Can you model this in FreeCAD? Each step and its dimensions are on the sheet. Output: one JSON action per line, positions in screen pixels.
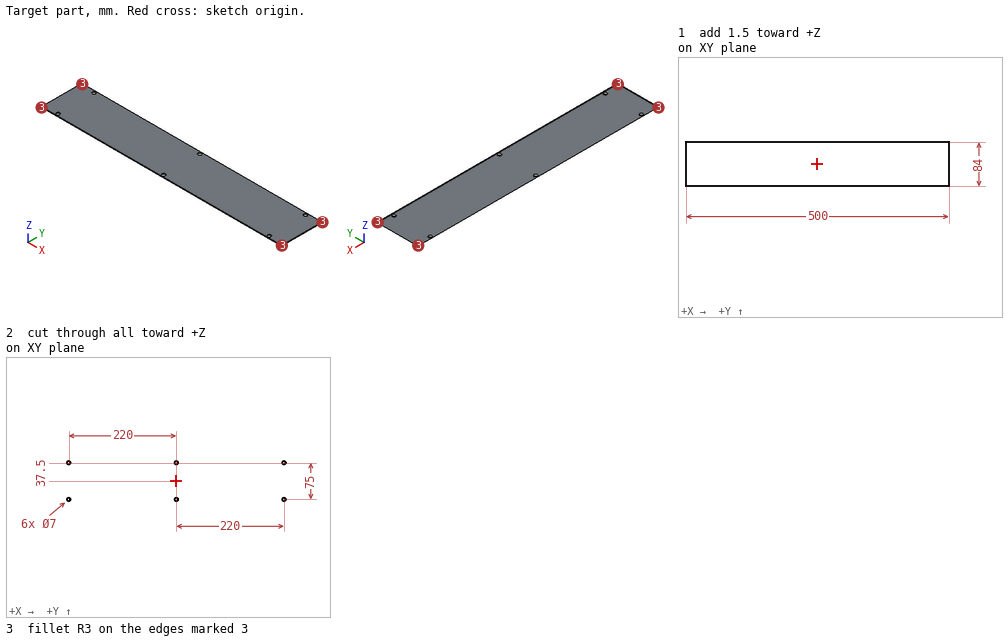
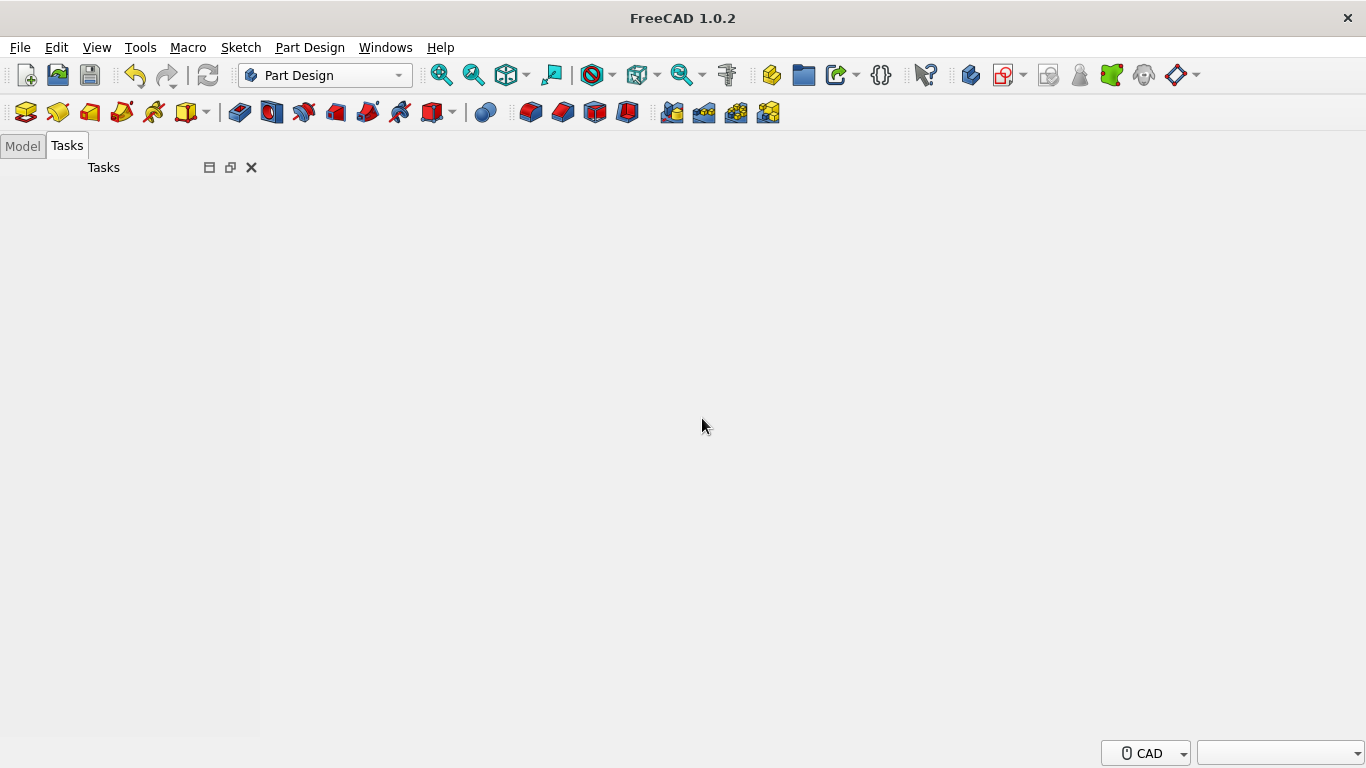
{"action": "left_click", "coordinate": [26, 76]}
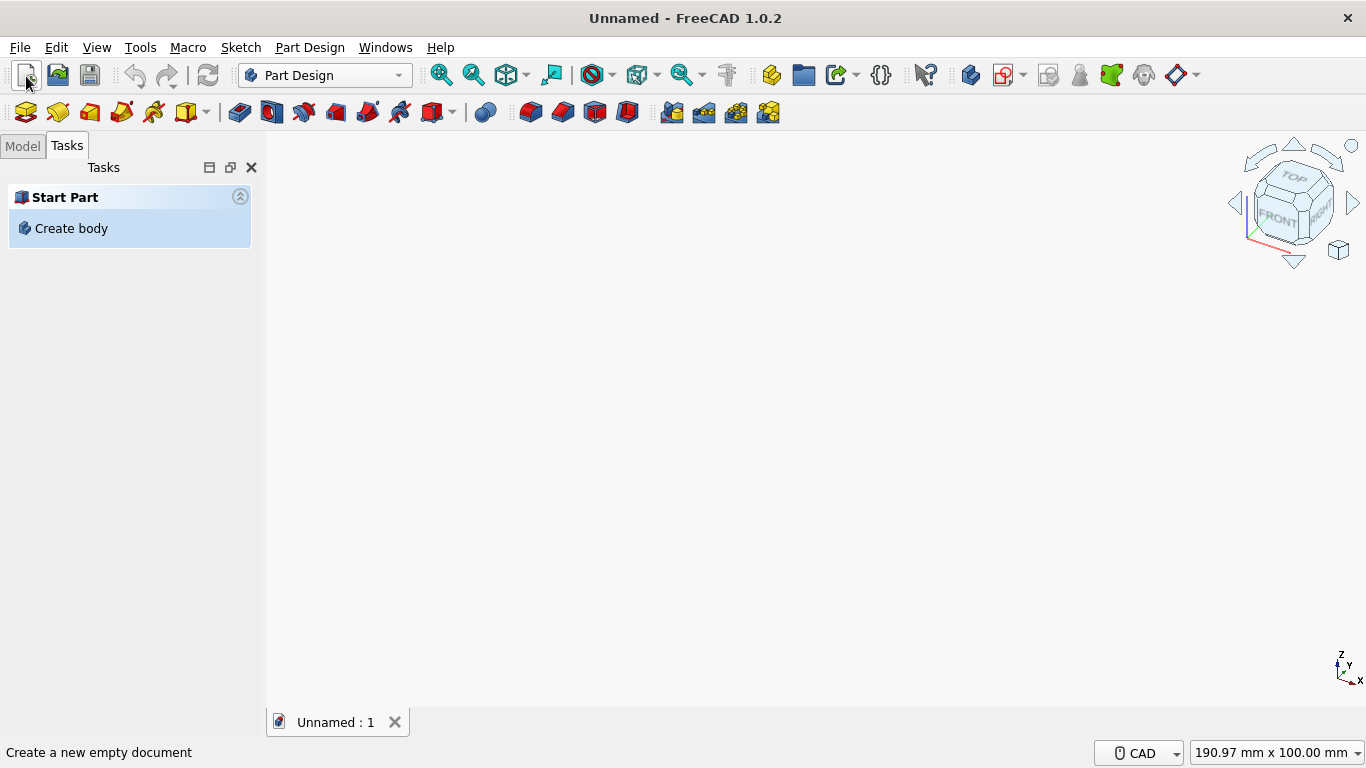
{"action": "left_click", "coordinate": [1004, 76]}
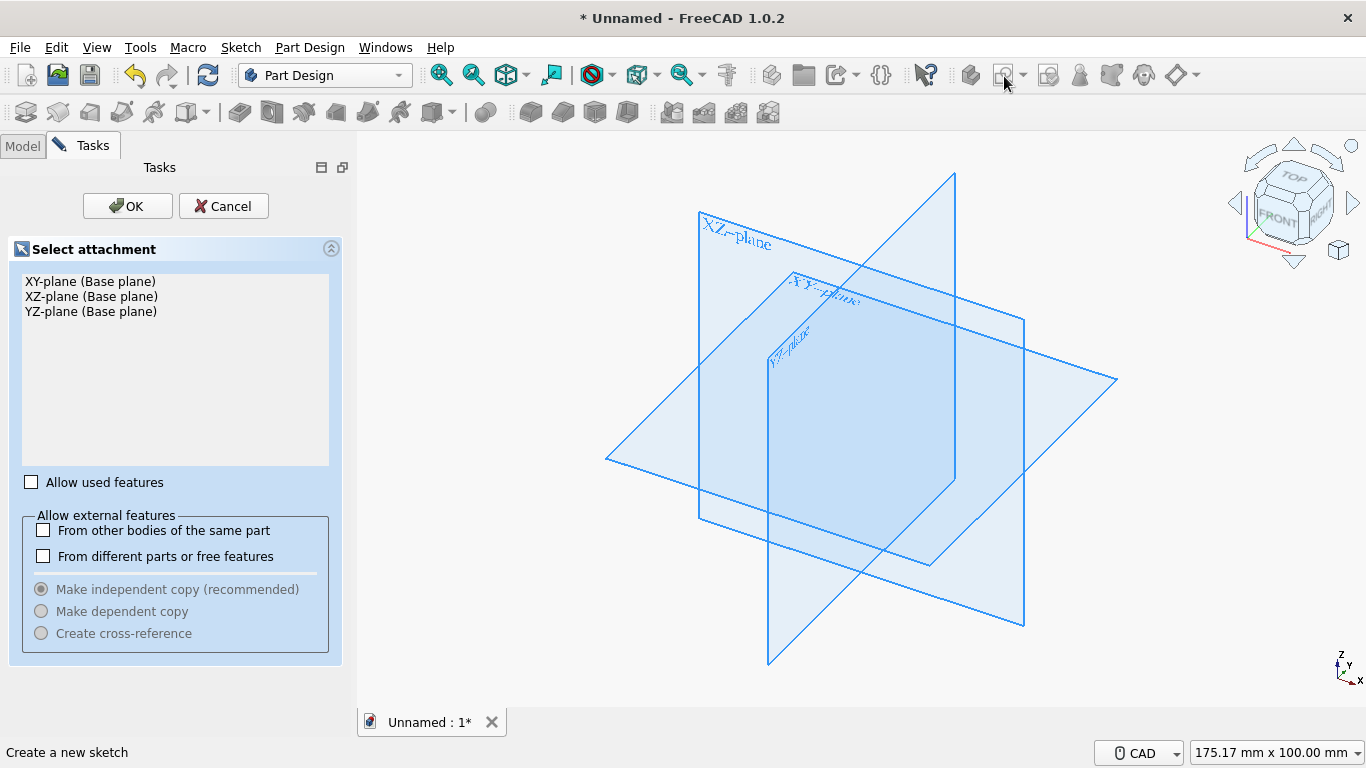
{"action": "left_click", "coordinate": [82, 282]}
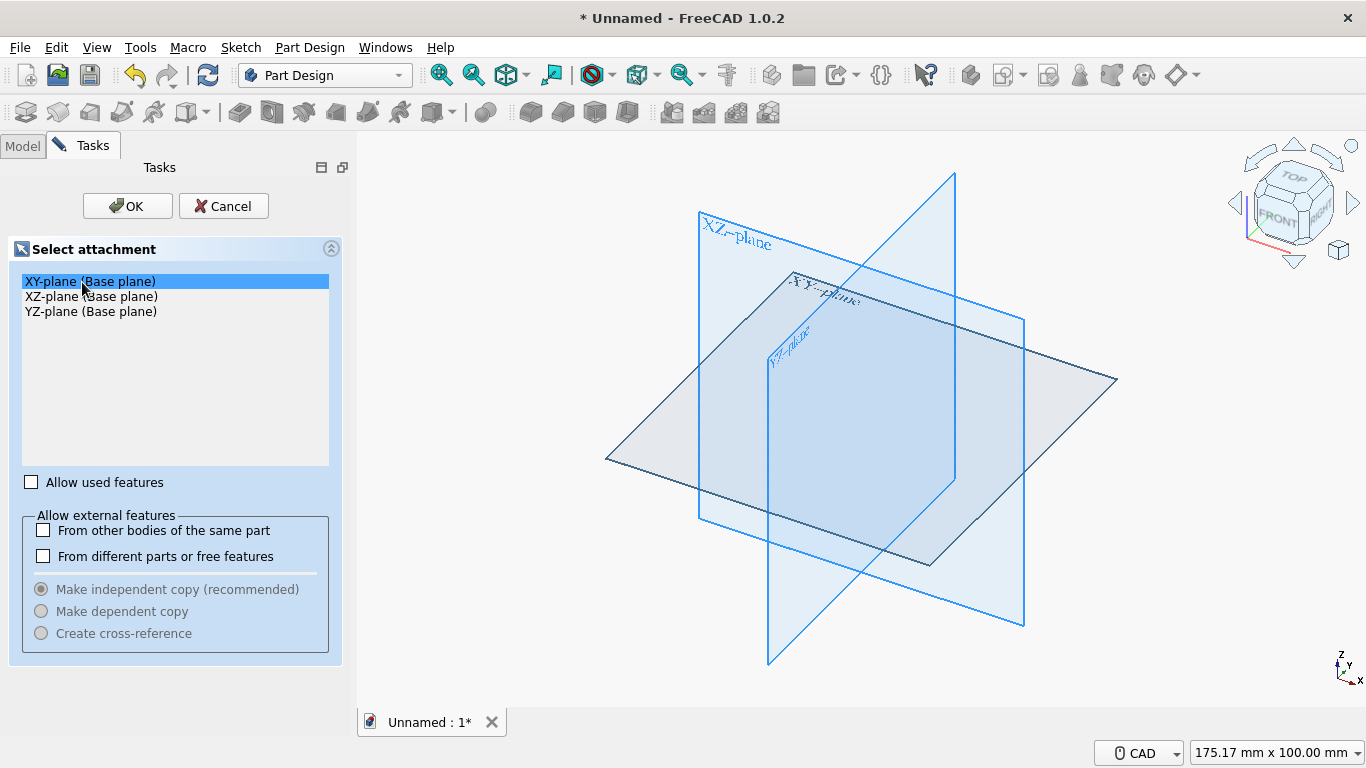
{"action": "left_click", "coordinate": [128, 206]}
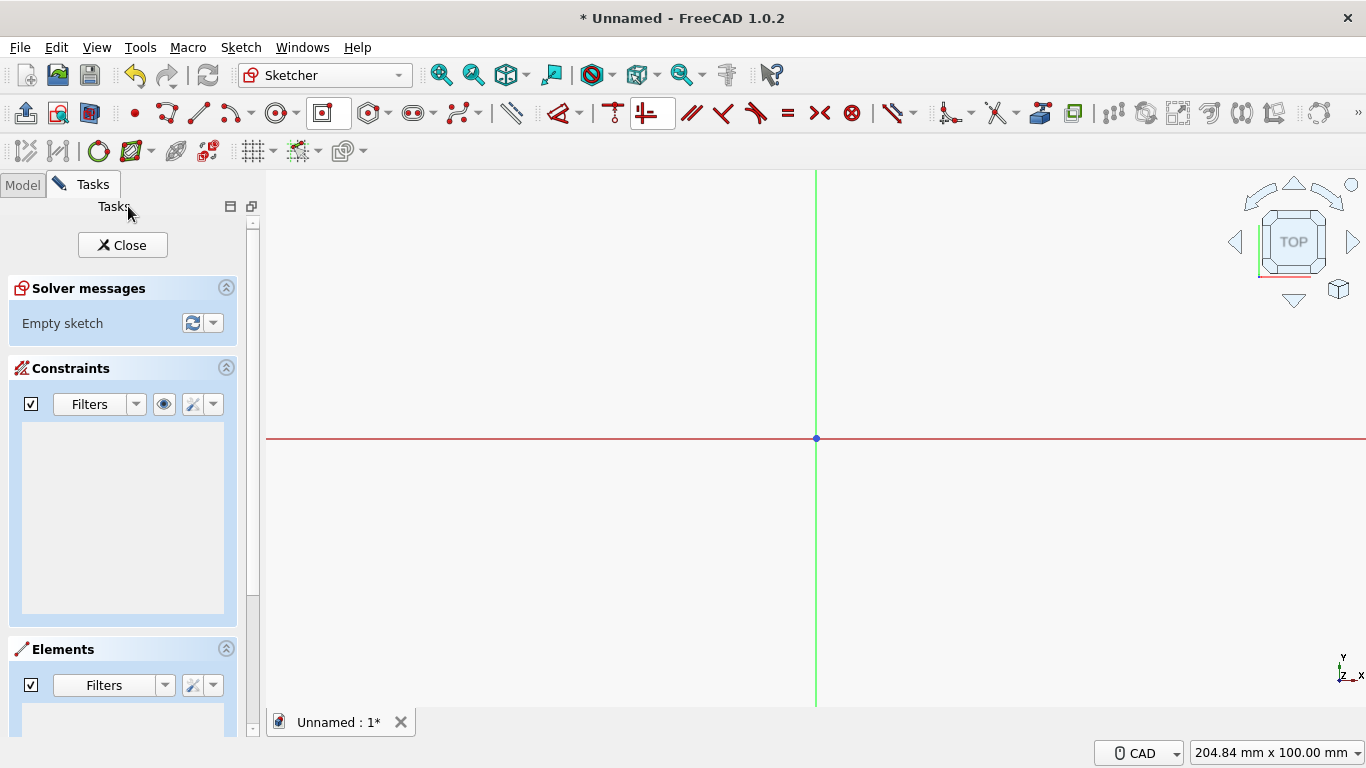
{"action": "scroll", "coordinate": [725, 438], "scroll_direction": "down", "scroll_amount": 7}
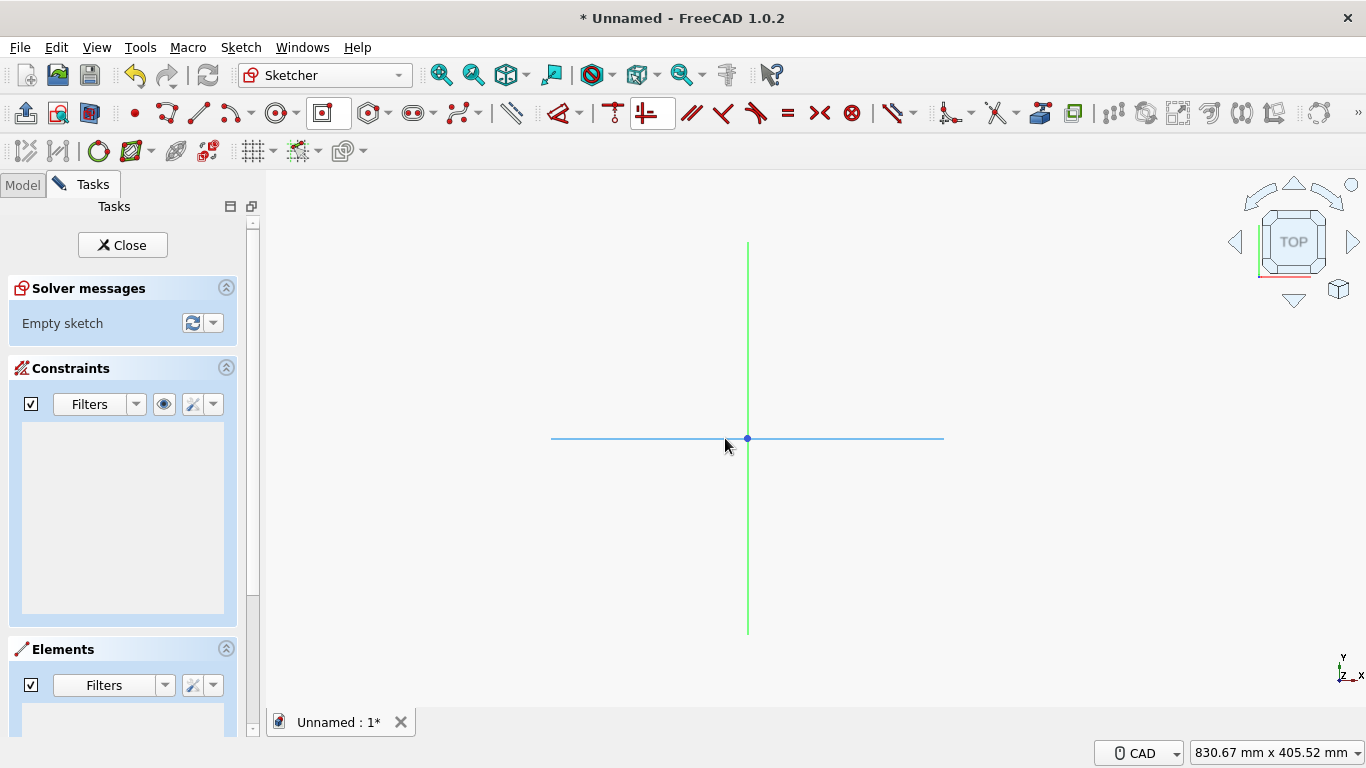
{"action": "left_click", "coordinate": [322, 114]}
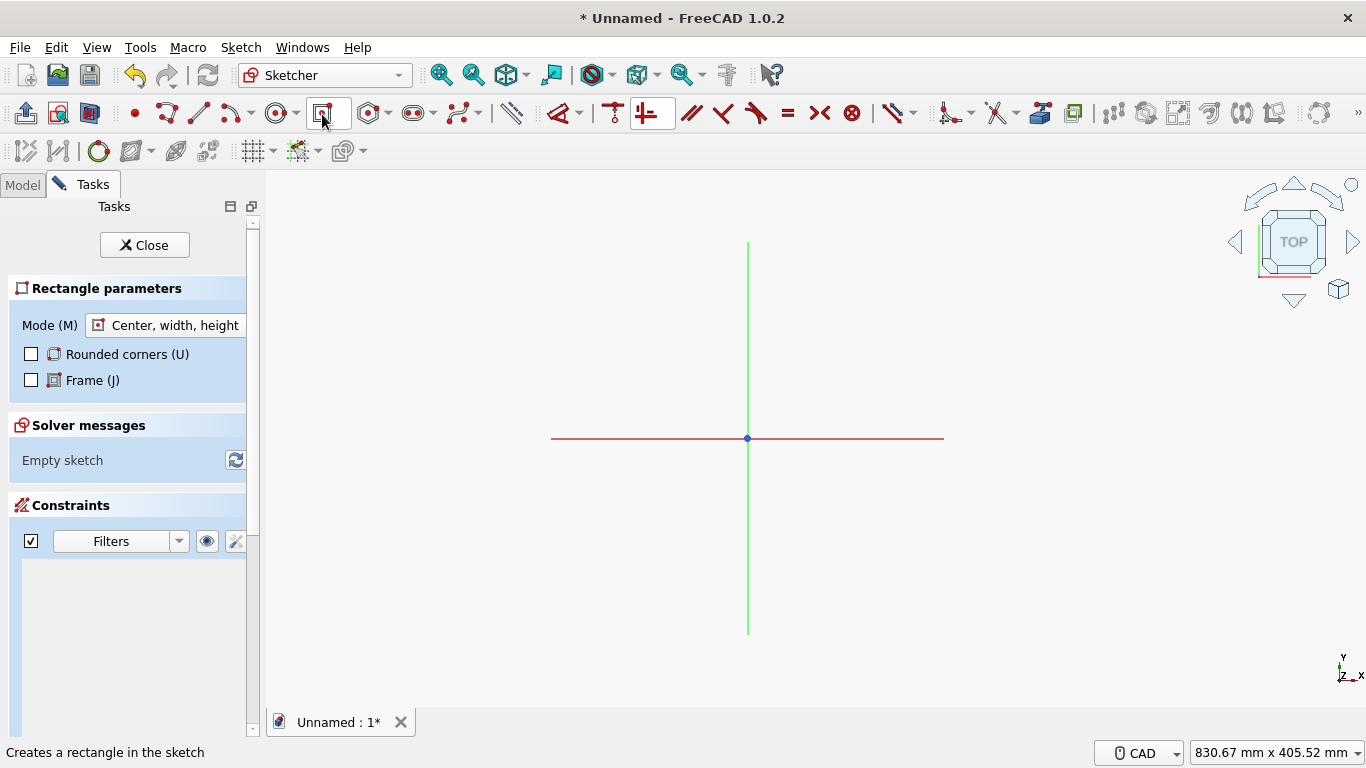
{"action": "left_click", "coordinate": [748, 438]}
{"action": "mouse_move", "coordinate": [1079, 383]}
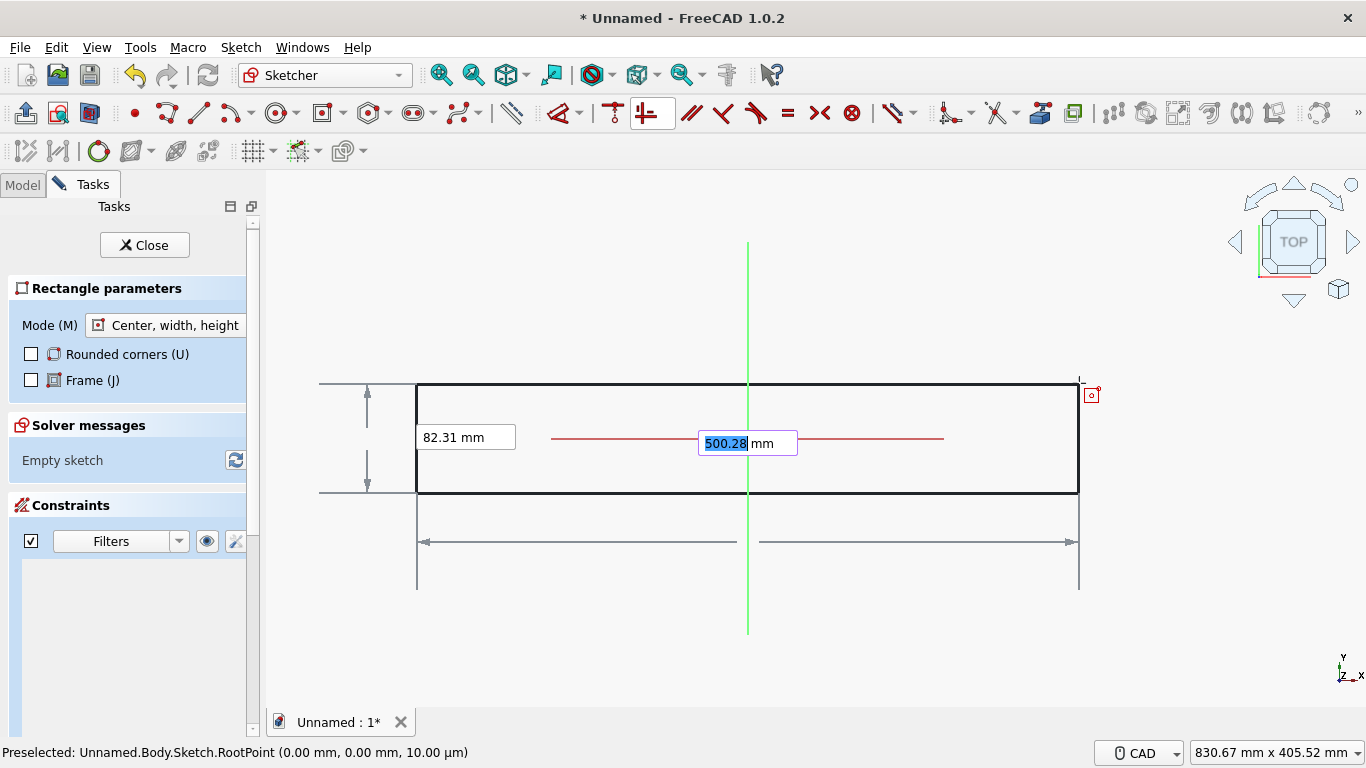
{"action": "type", "text": "500"}
{"action": "key", "text": "Tab"}
{"action": "type", "text": "84"}
{"action": "key", "text": "Return"}
{"action": "key", "text": "Escape"}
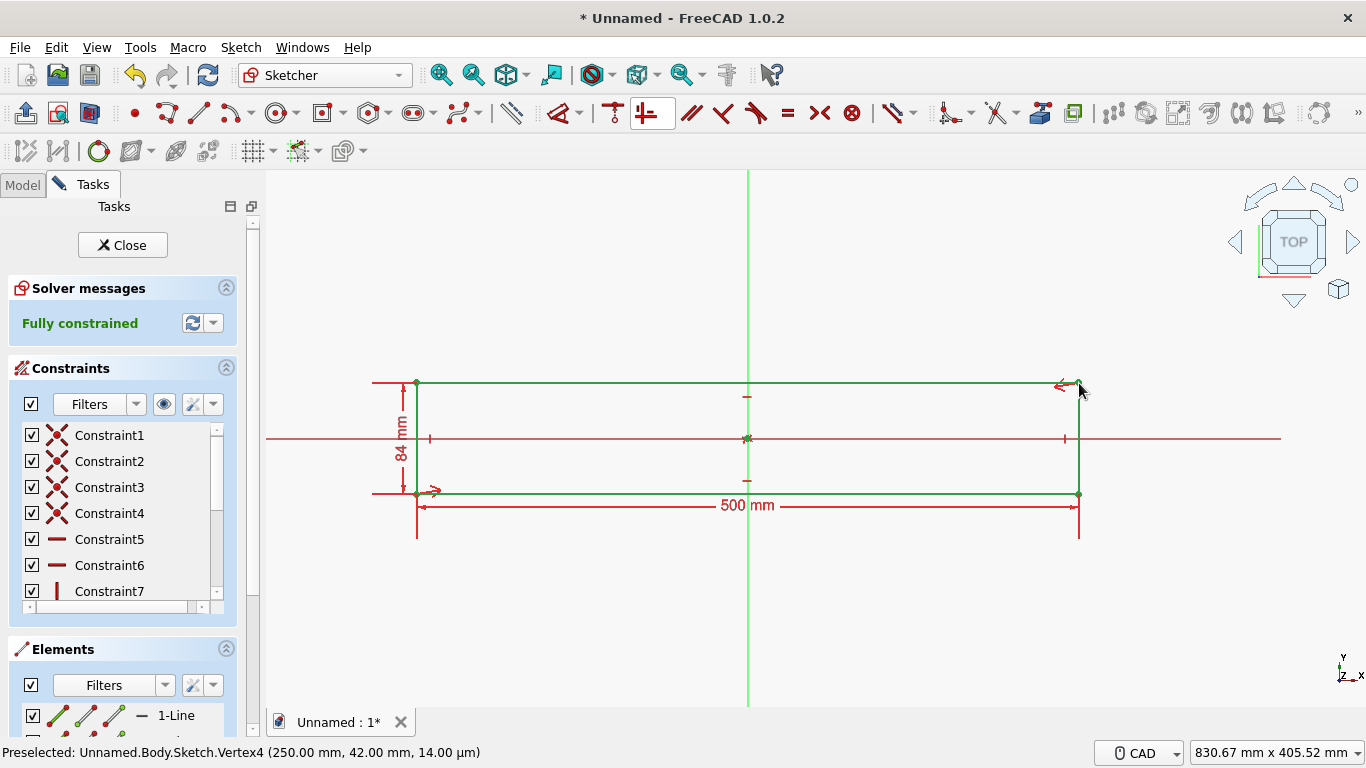
{"action": "left_click", "coordinate": [123, 245]}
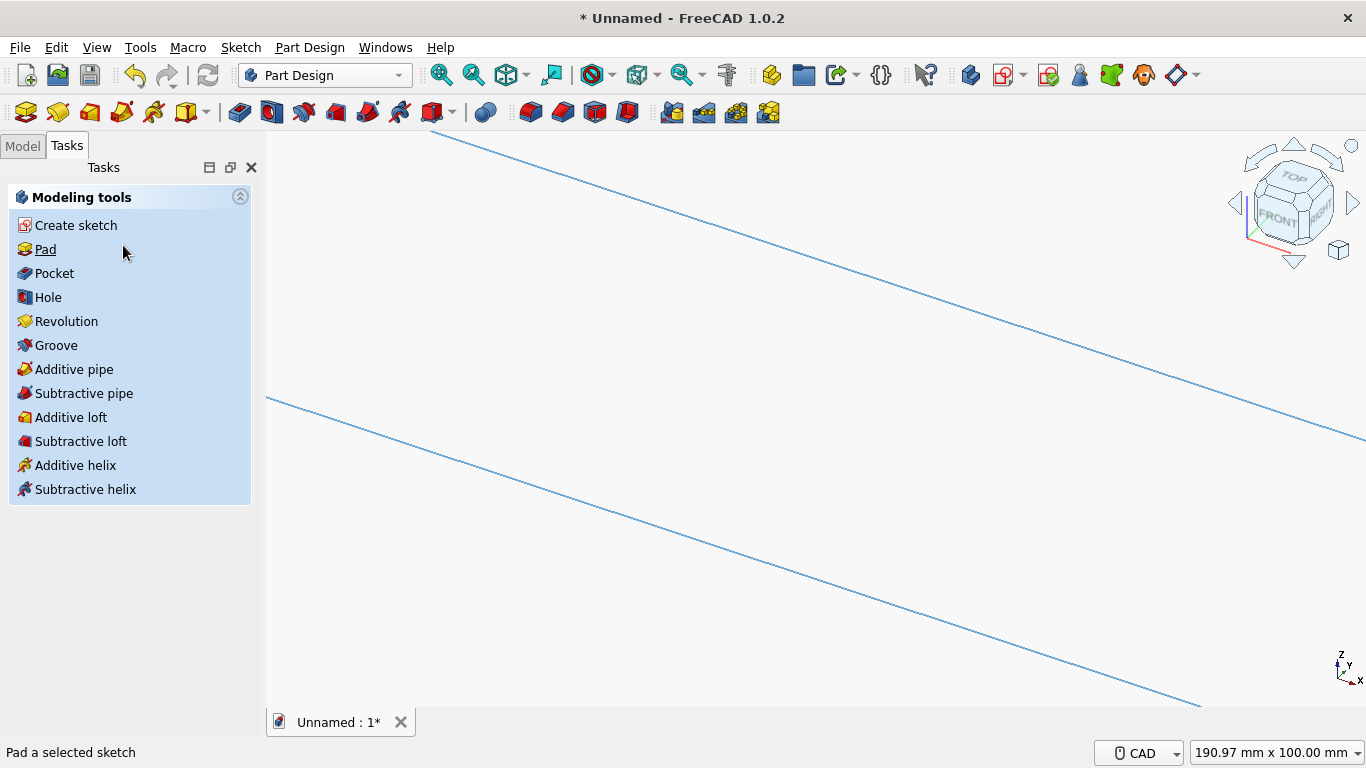
{"action": "left_click", "coordinate": [26, 112]}